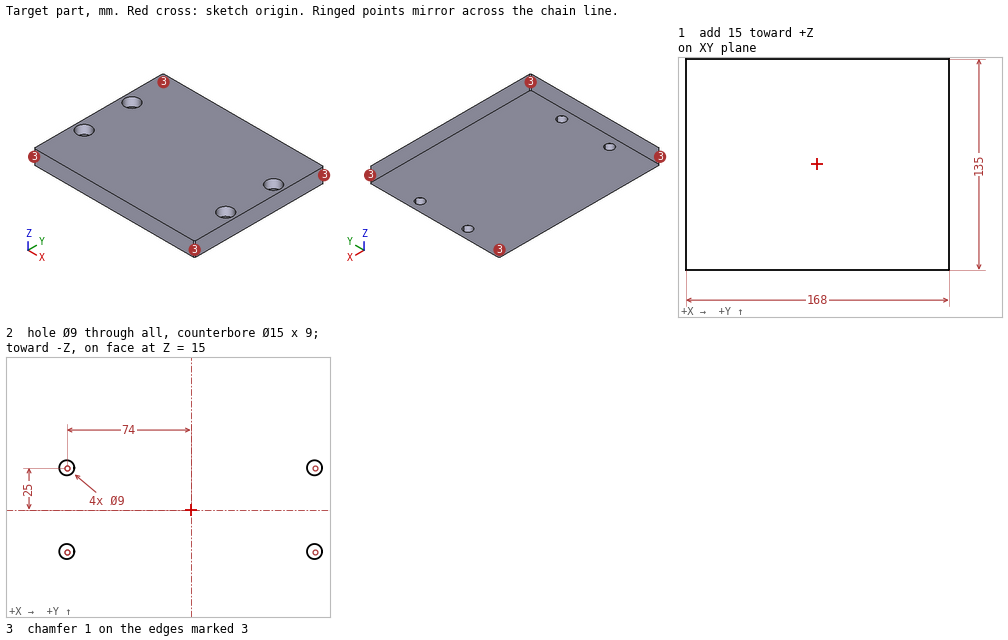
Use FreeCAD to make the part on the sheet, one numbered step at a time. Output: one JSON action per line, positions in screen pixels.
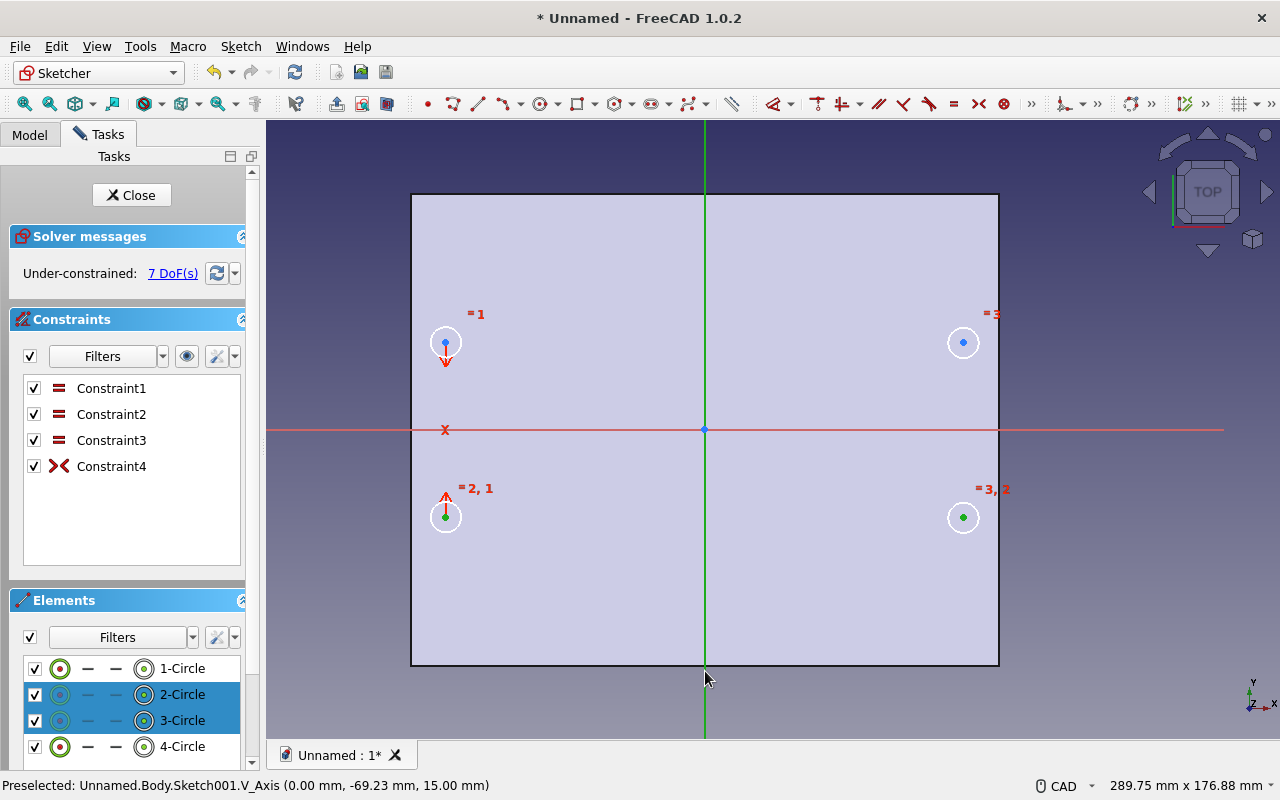
{"action": "left_click", "coordinate": [979, 104]}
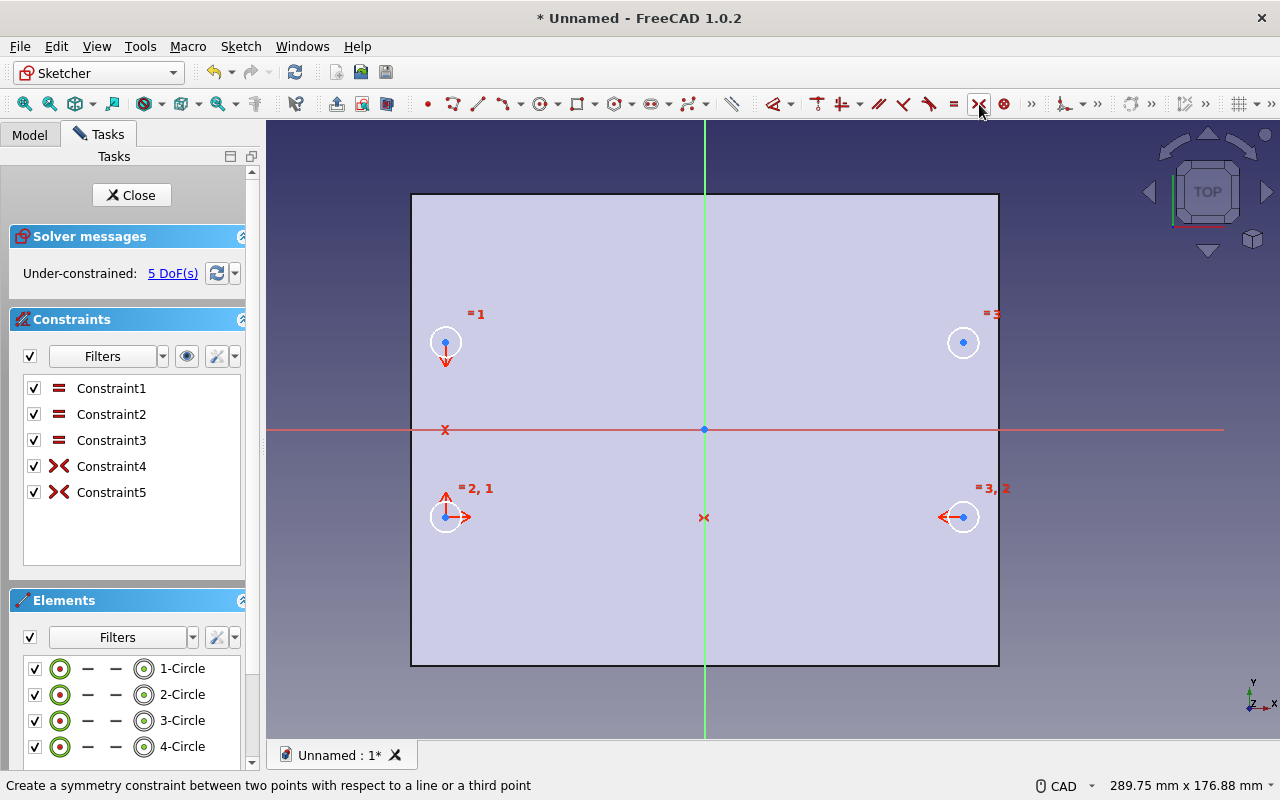
{"action": "left_click", "coordinate": [446, 342]}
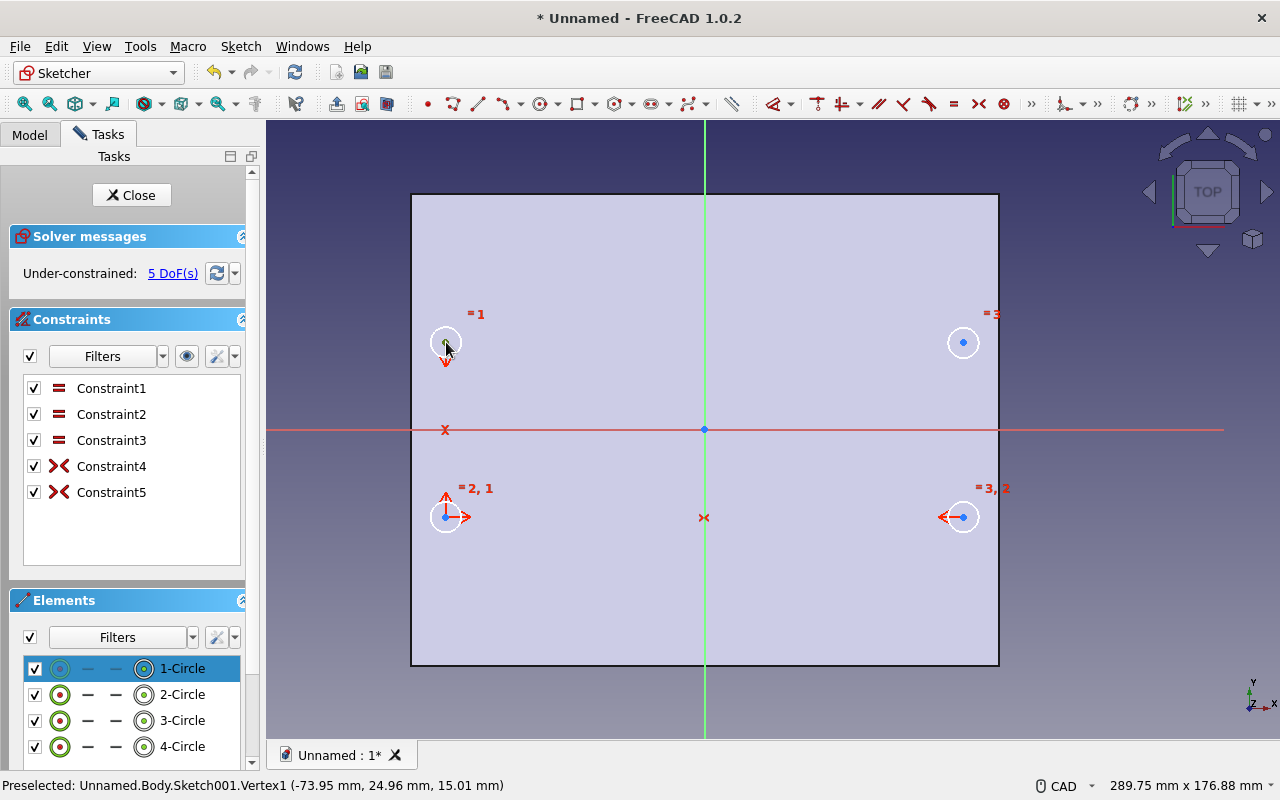
{"action": "left_click", "coordinate": [964, 343]}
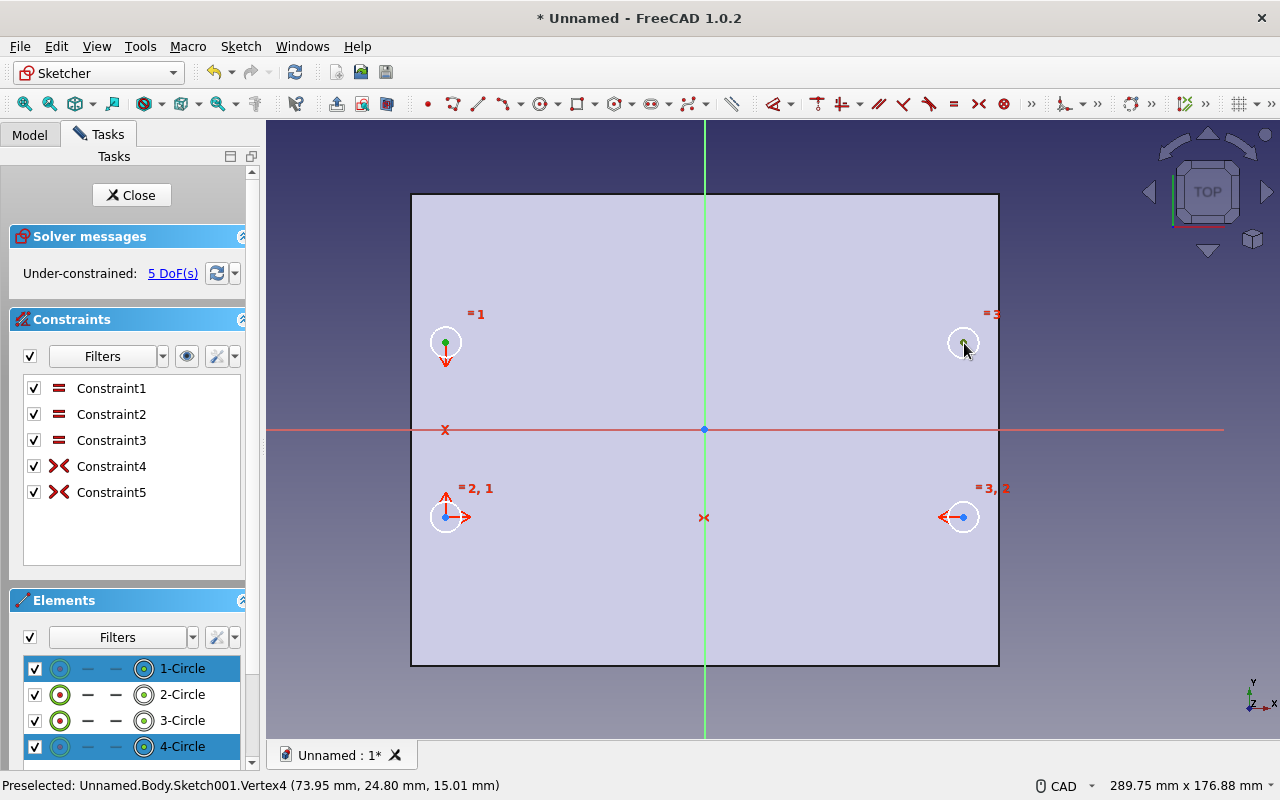
{"action": "left_click", "coordinate": [705, 671]}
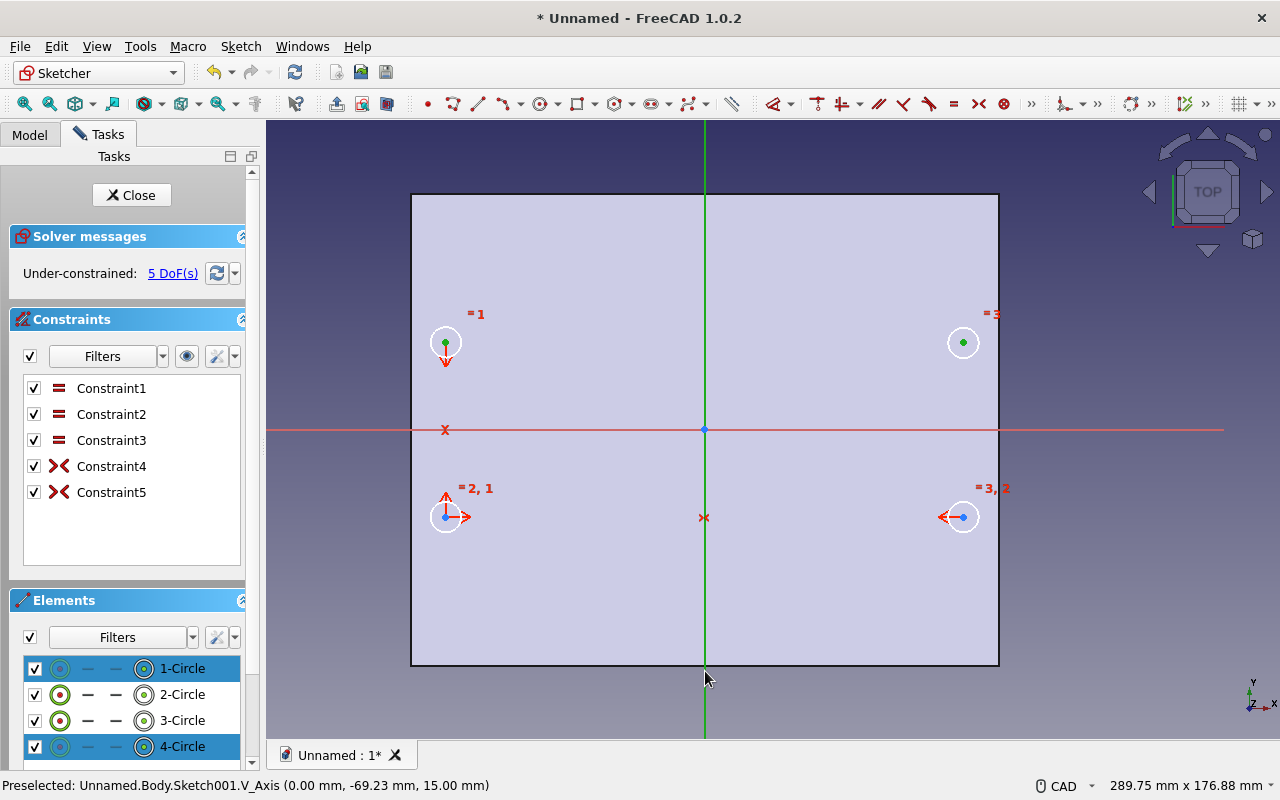
{"action": "left_click", "coordinate": [979, 104]}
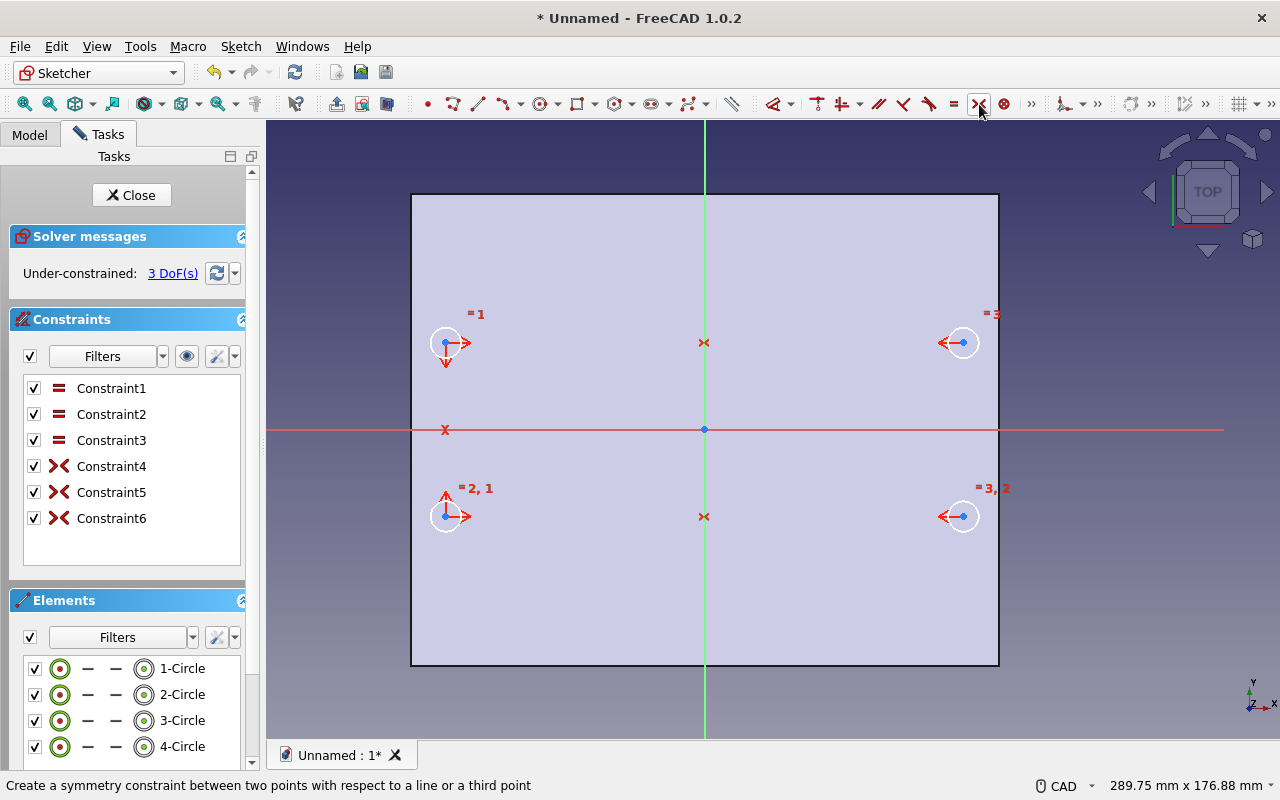
{"action": "left_click", "coordinate": [772, 104]}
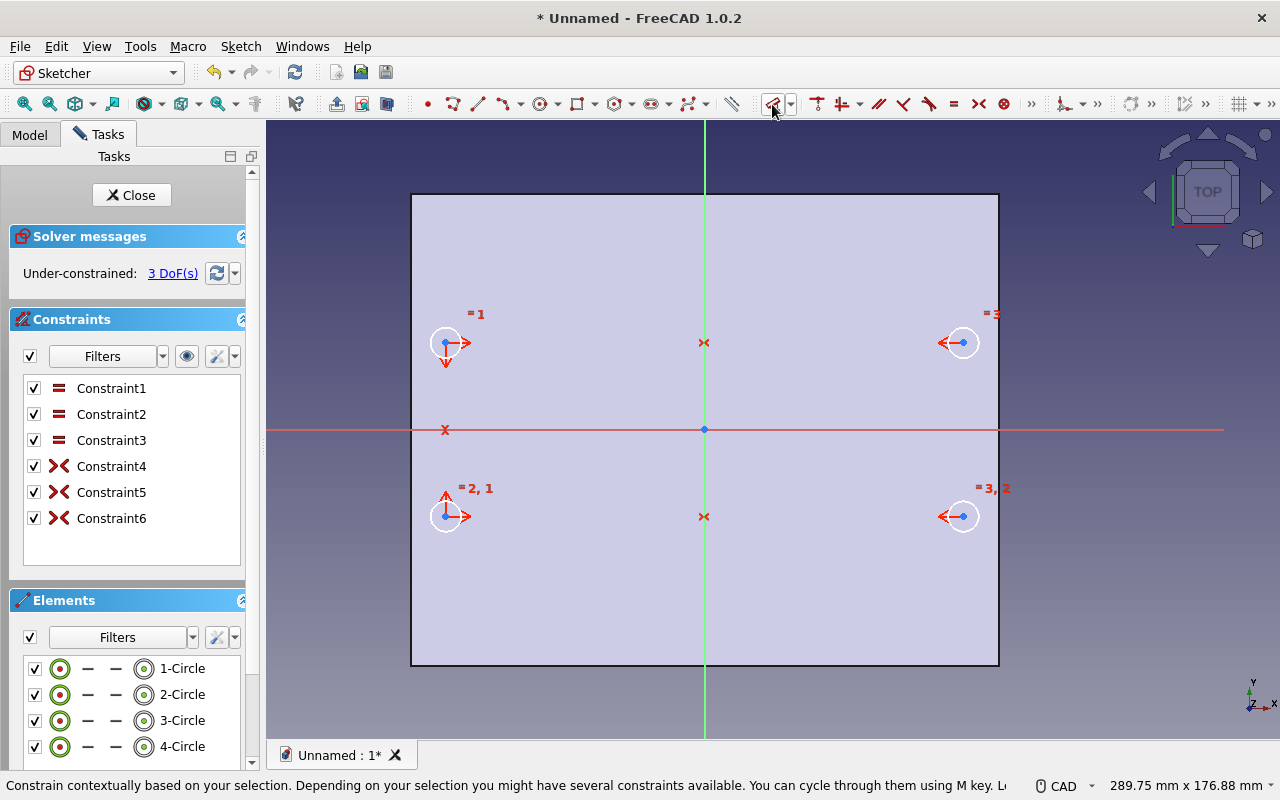
{"action": "scroll", "coordinate": [457, 332], "scroll_direction": "up", "scroll_amount": 2}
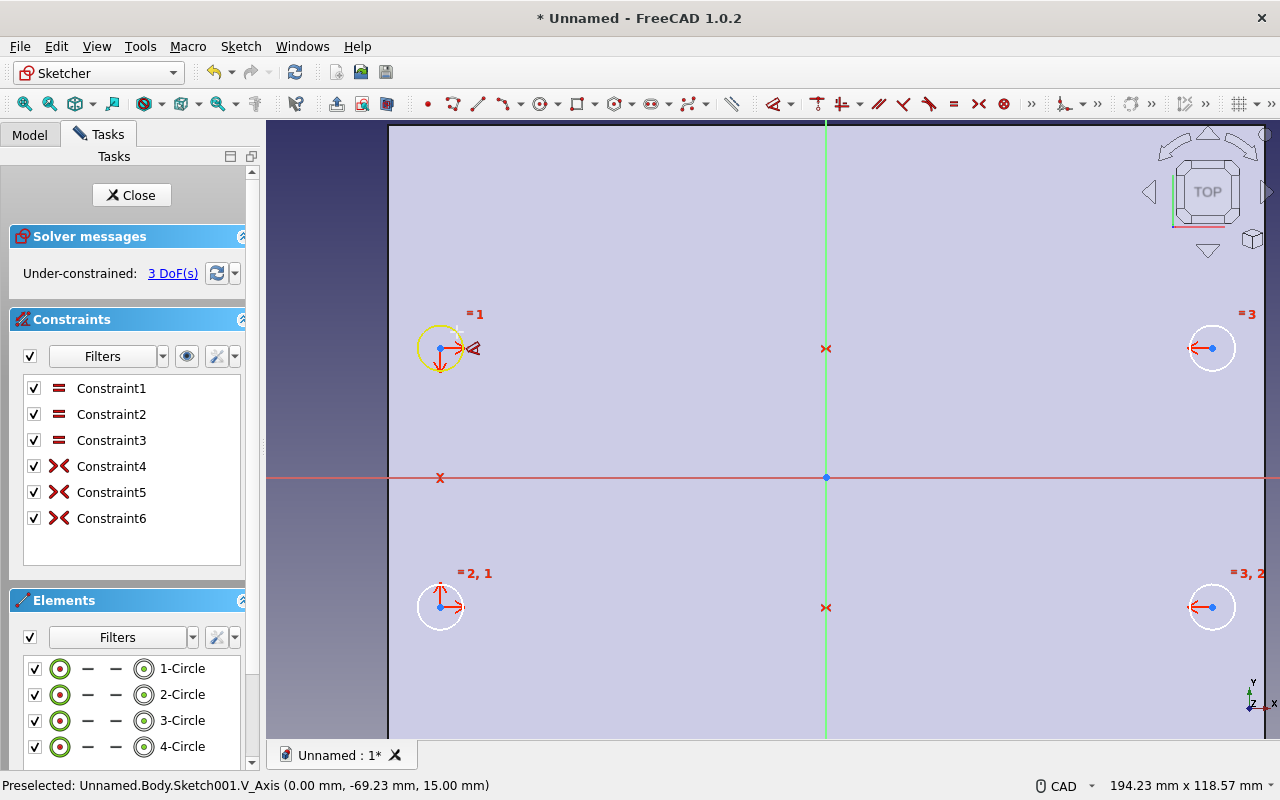
{"action": "left_click", "coordinate": [456, 332]}
{"action": "left_click", "coordinate": [478, 309]}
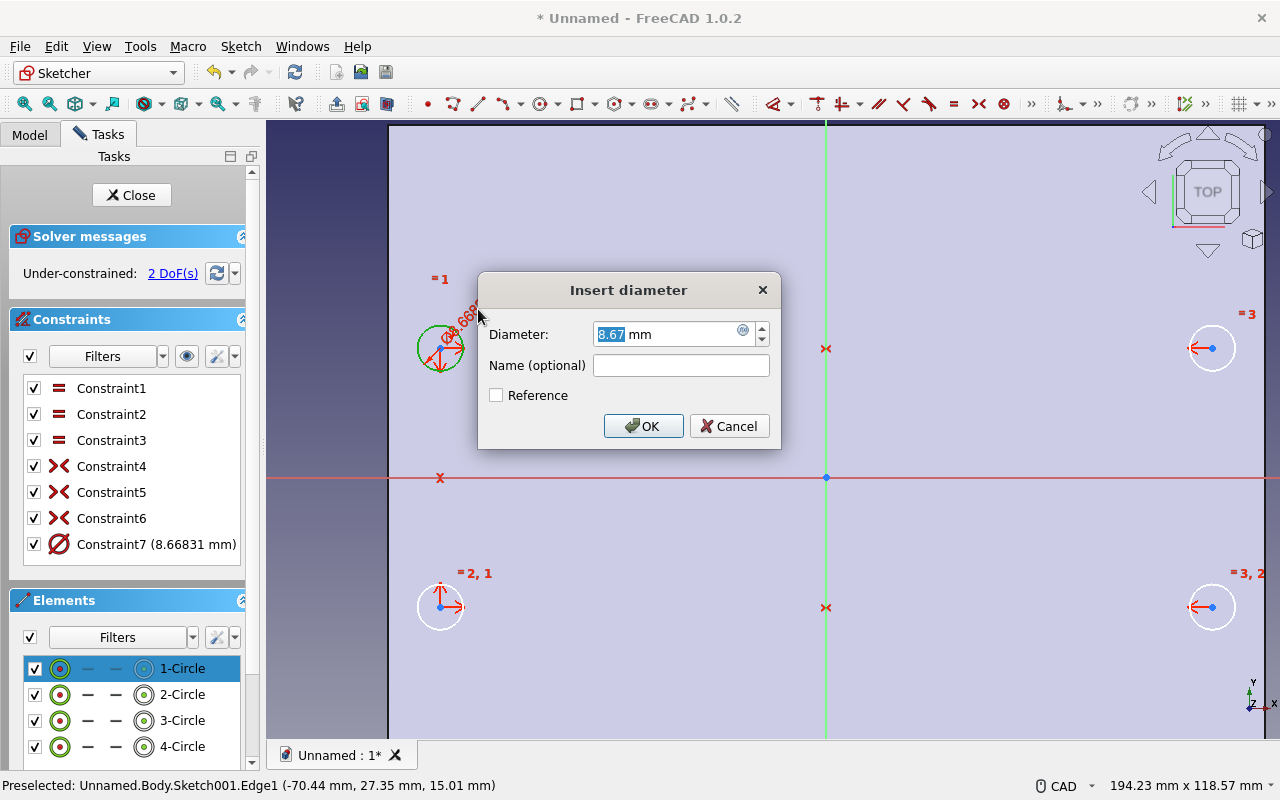
{"action": "type", "text": "9"}
{"action": "key", "text": "Return"}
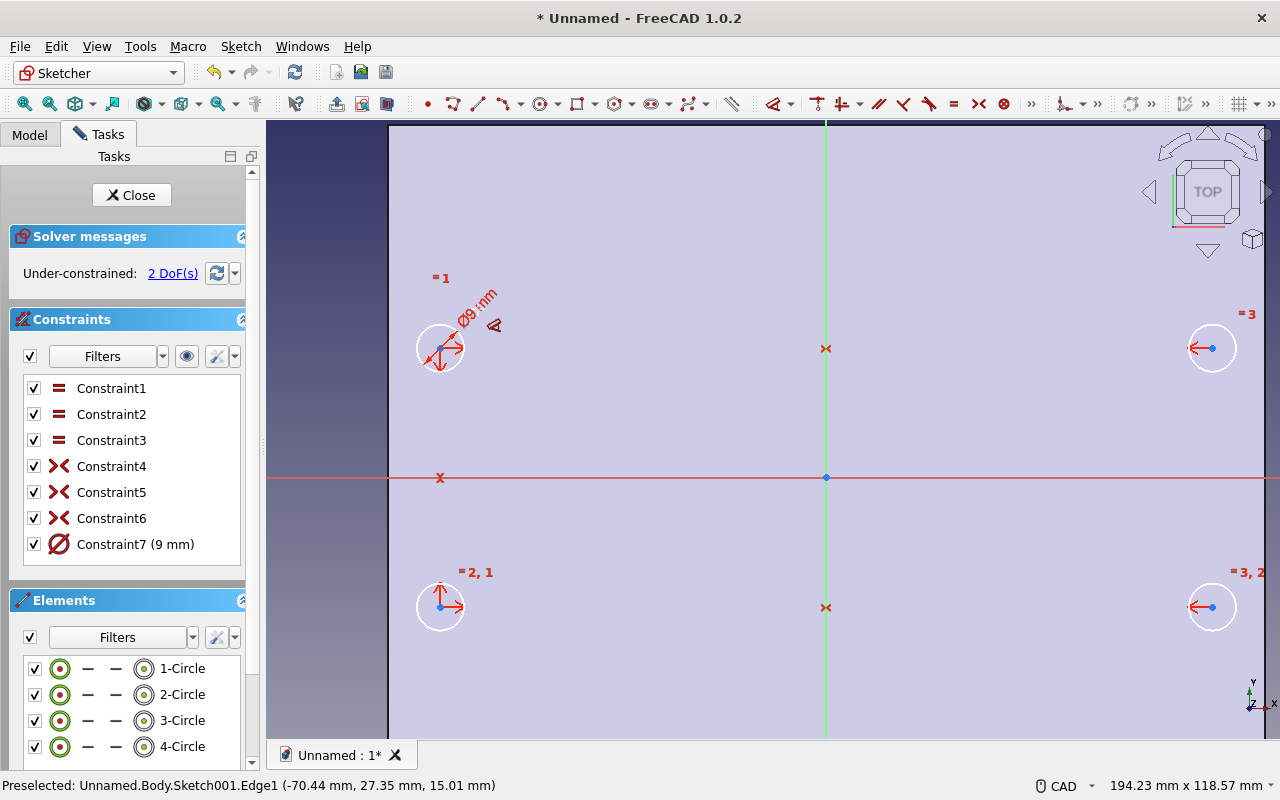
{"action": "left_click", "coordinate": [440, 348]}
{"action": "left_click", "coordinate": [633, 314]}